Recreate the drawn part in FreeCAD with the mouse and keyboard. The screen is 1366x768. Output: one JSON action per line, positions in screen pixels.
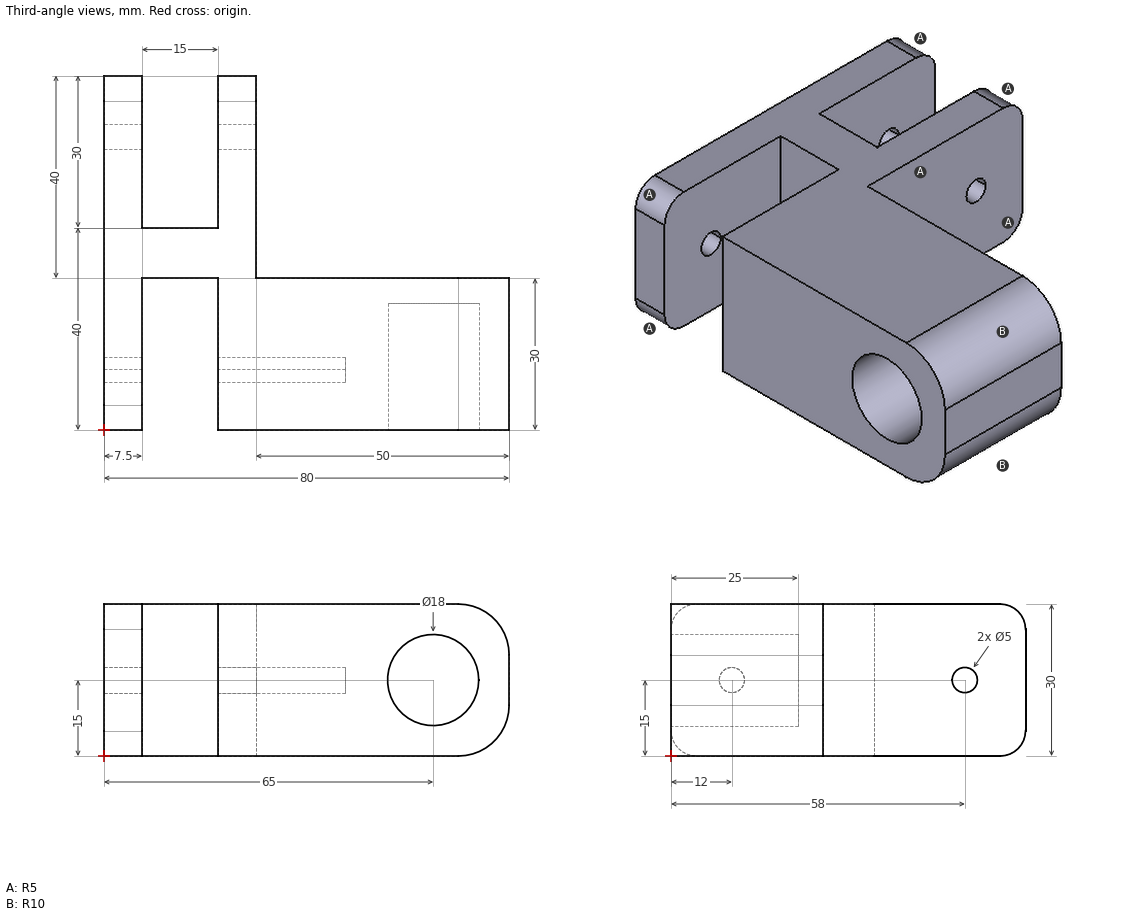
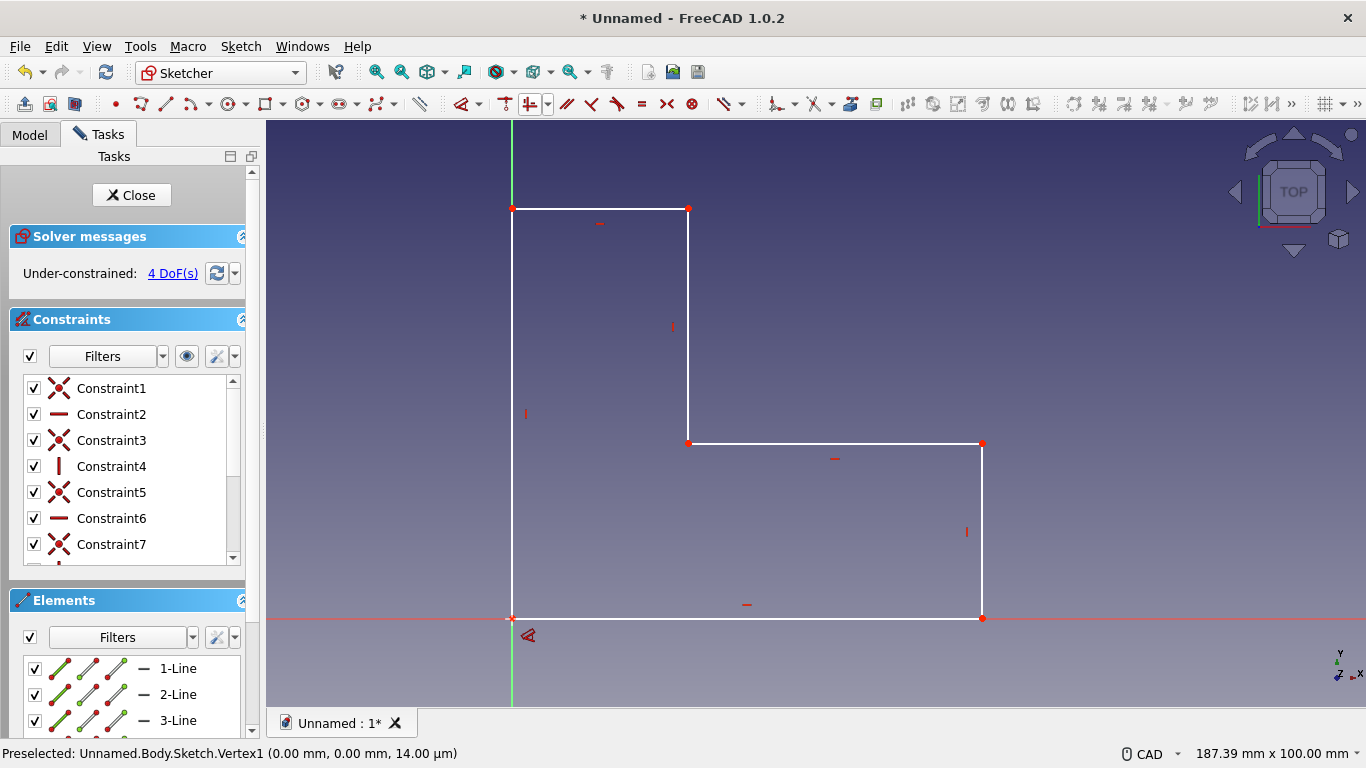
{"action": "left_click", "coordinate": [653, 619]}
{"action": "left_click", "coordinate": [747, 653]}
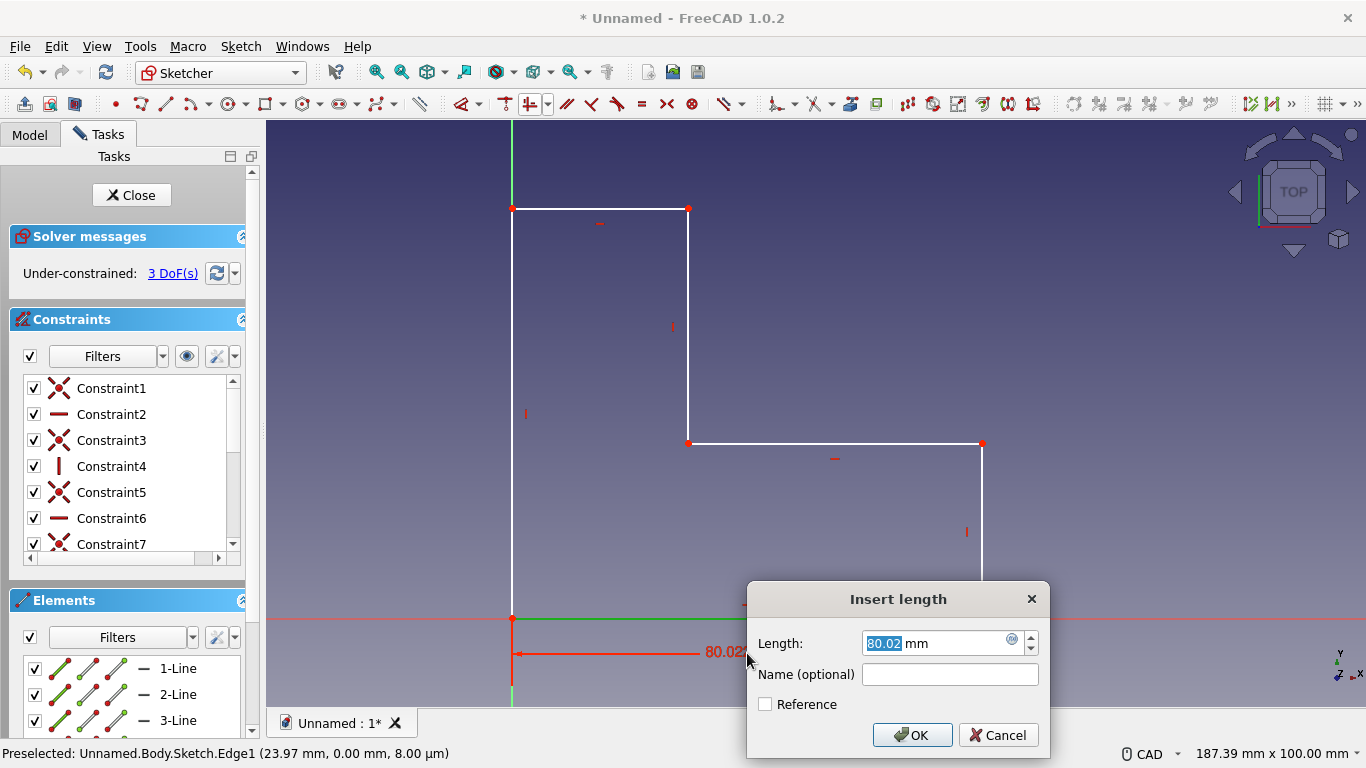
{"action": "type", "text": "80"}
{"action": "key", "text": "Return"}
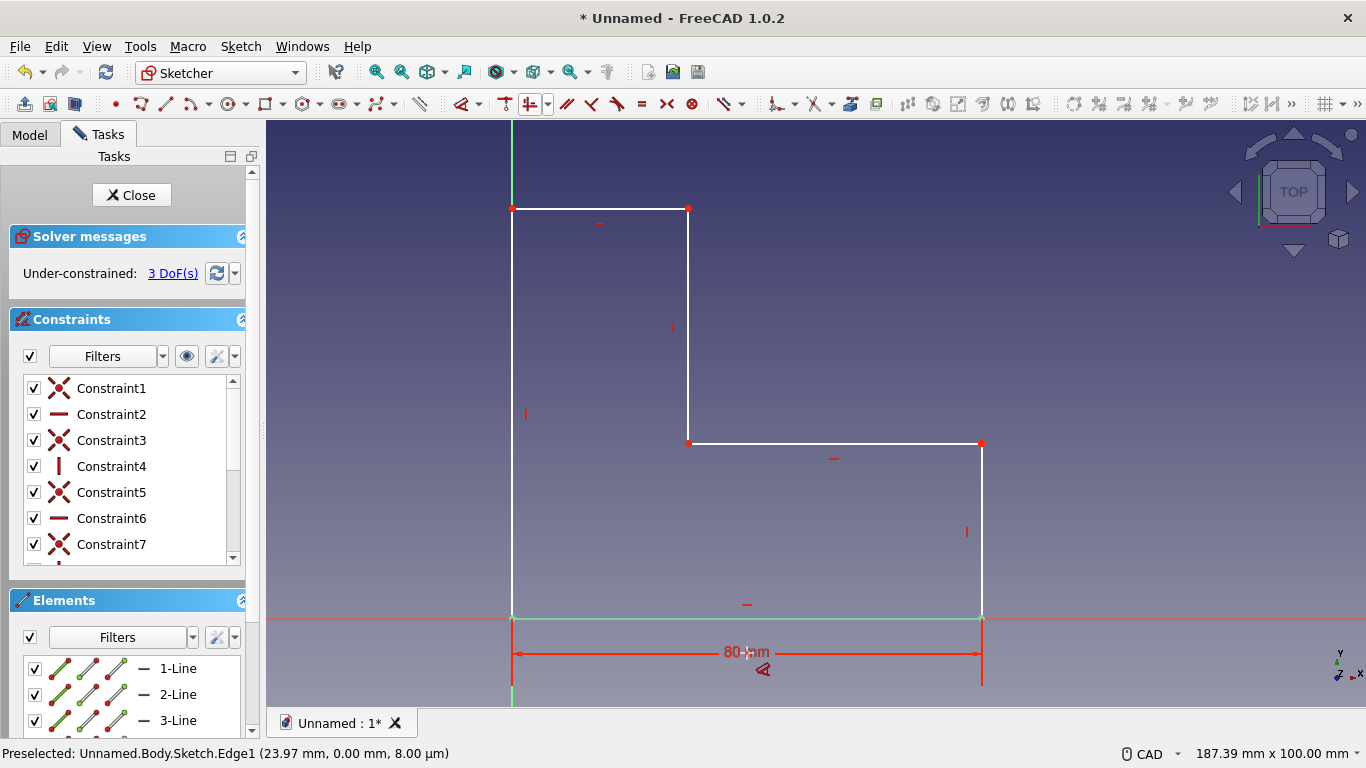
{"action": "left_click", "coordinate": [982, 566]}
{"action": "left_click", "coordinate": [1016, 531]}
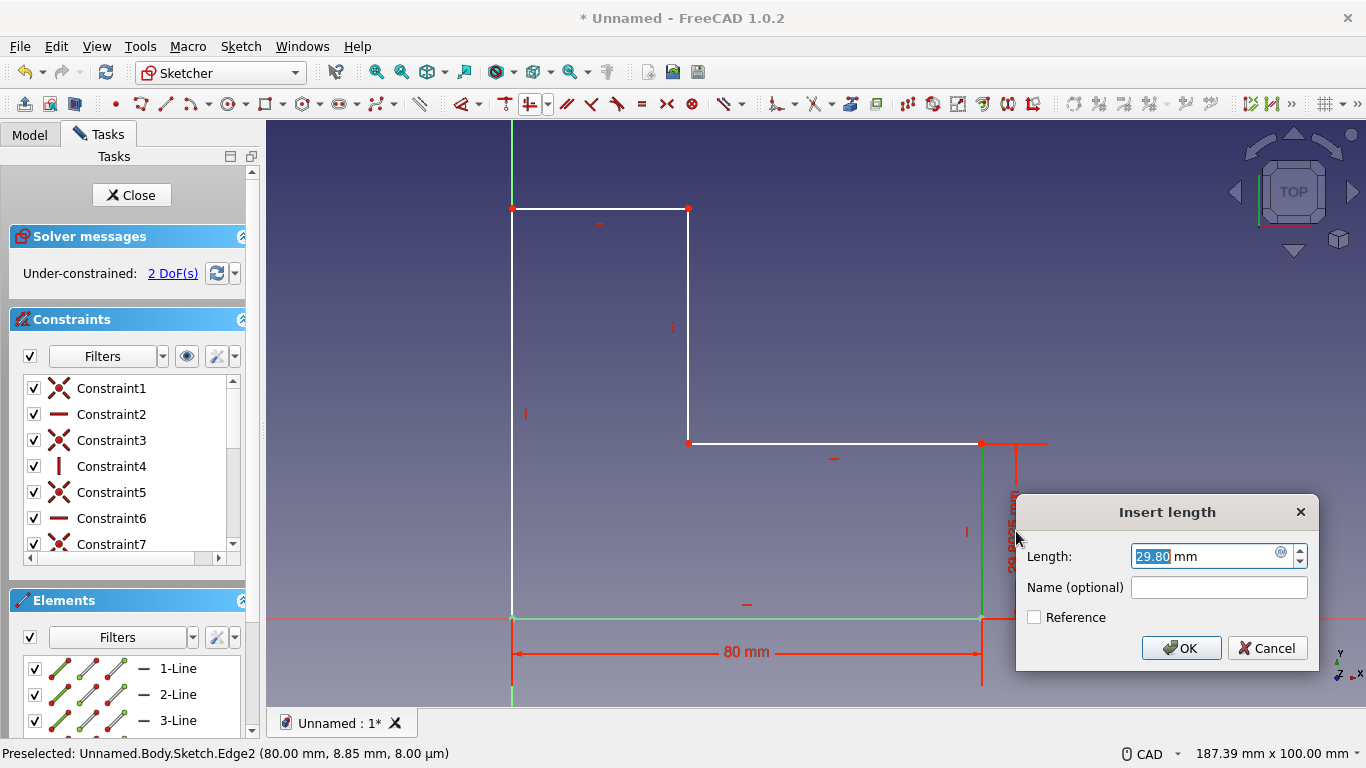
{"action": "type", "text": "30"}
{"action": "key", "text": "Return"}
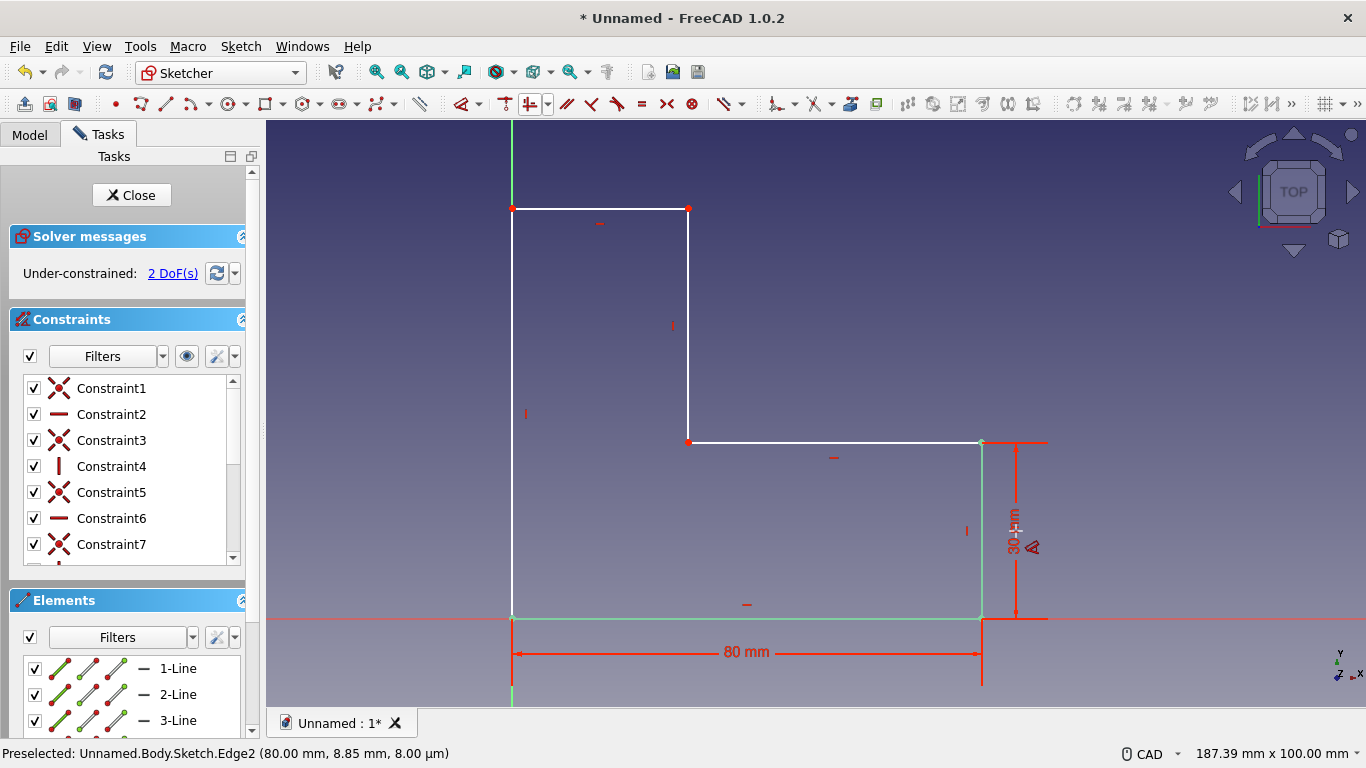
{"action": "left_click", "coordinate": [894, 443]}
{"action": "left_click", "coordinate": [835, 477]}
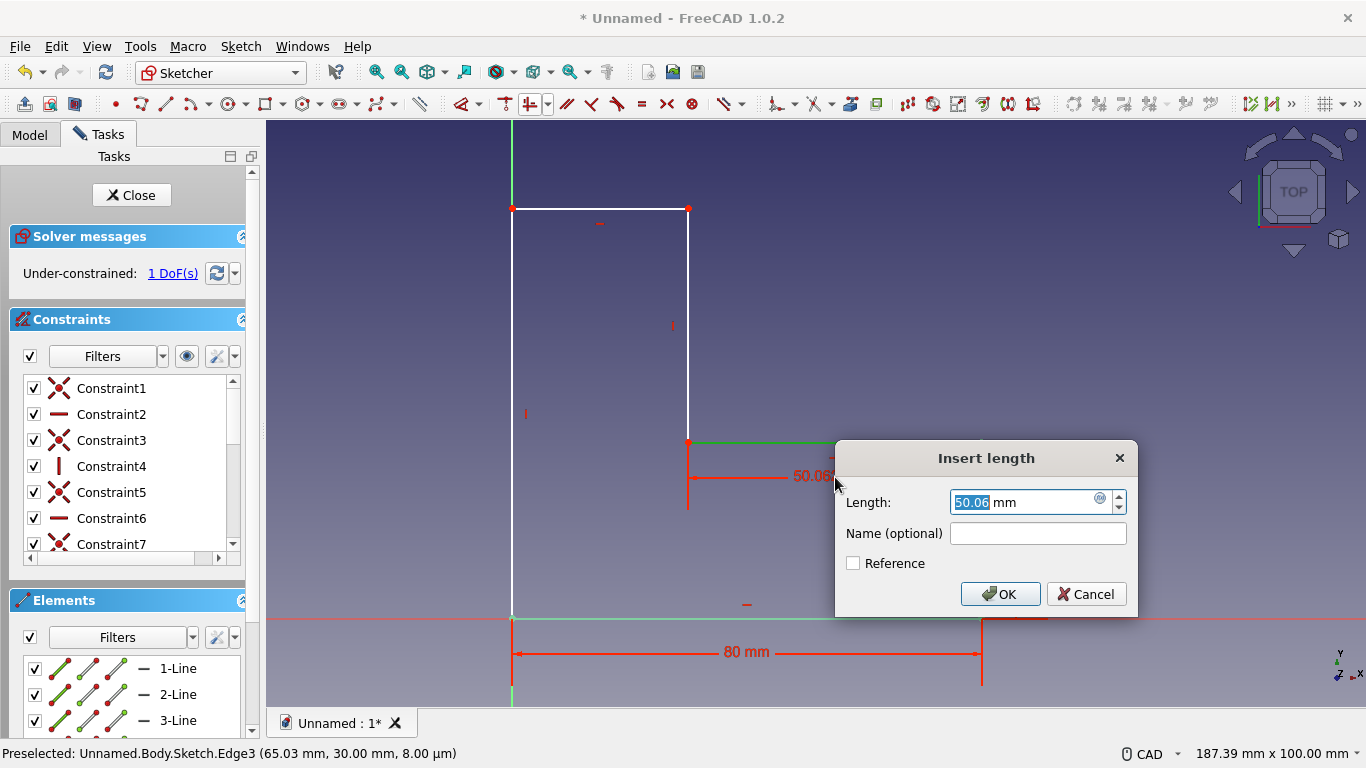
{"action": "type", "text": "50"}
{"action": "key", "text": "Return"}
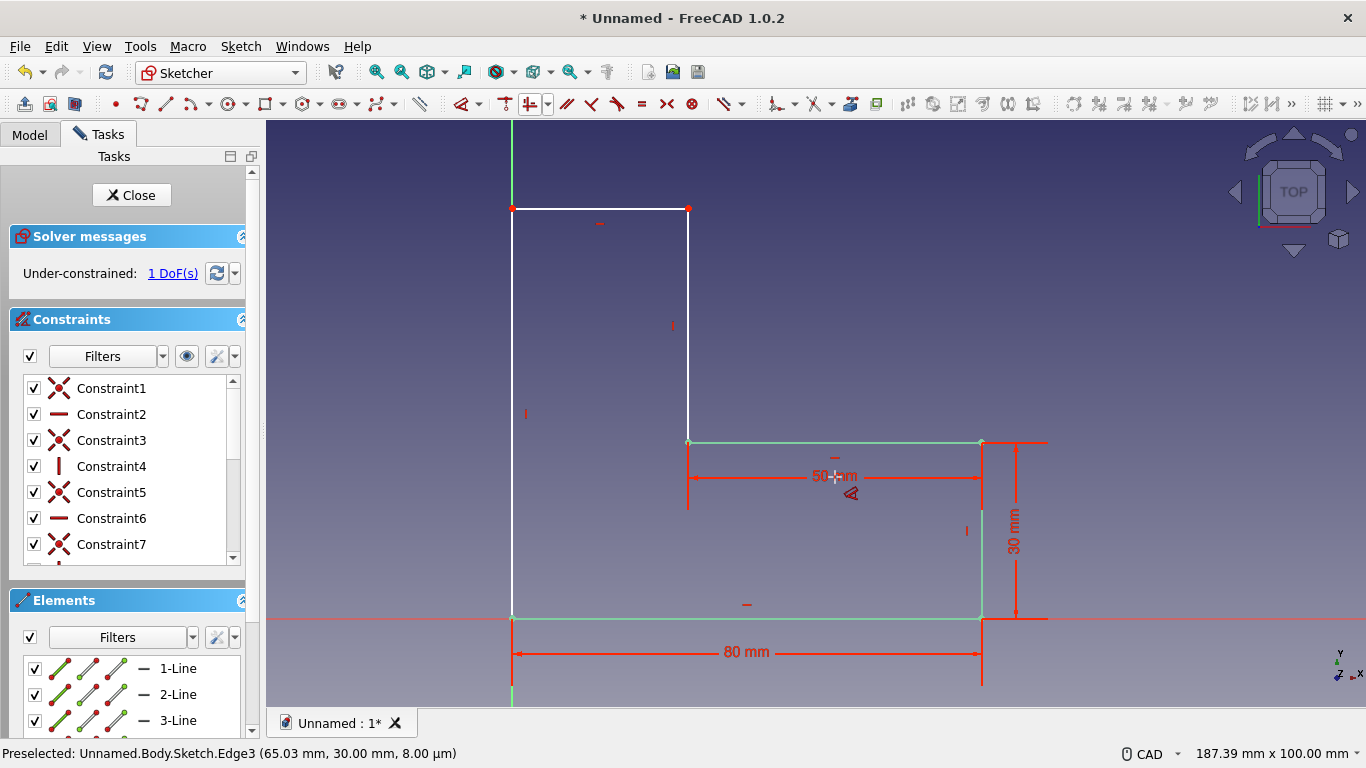
{"action": "left_click", "coordinate": [688, 373]}
{"action": "left_click", "coordinate": [654, 326]}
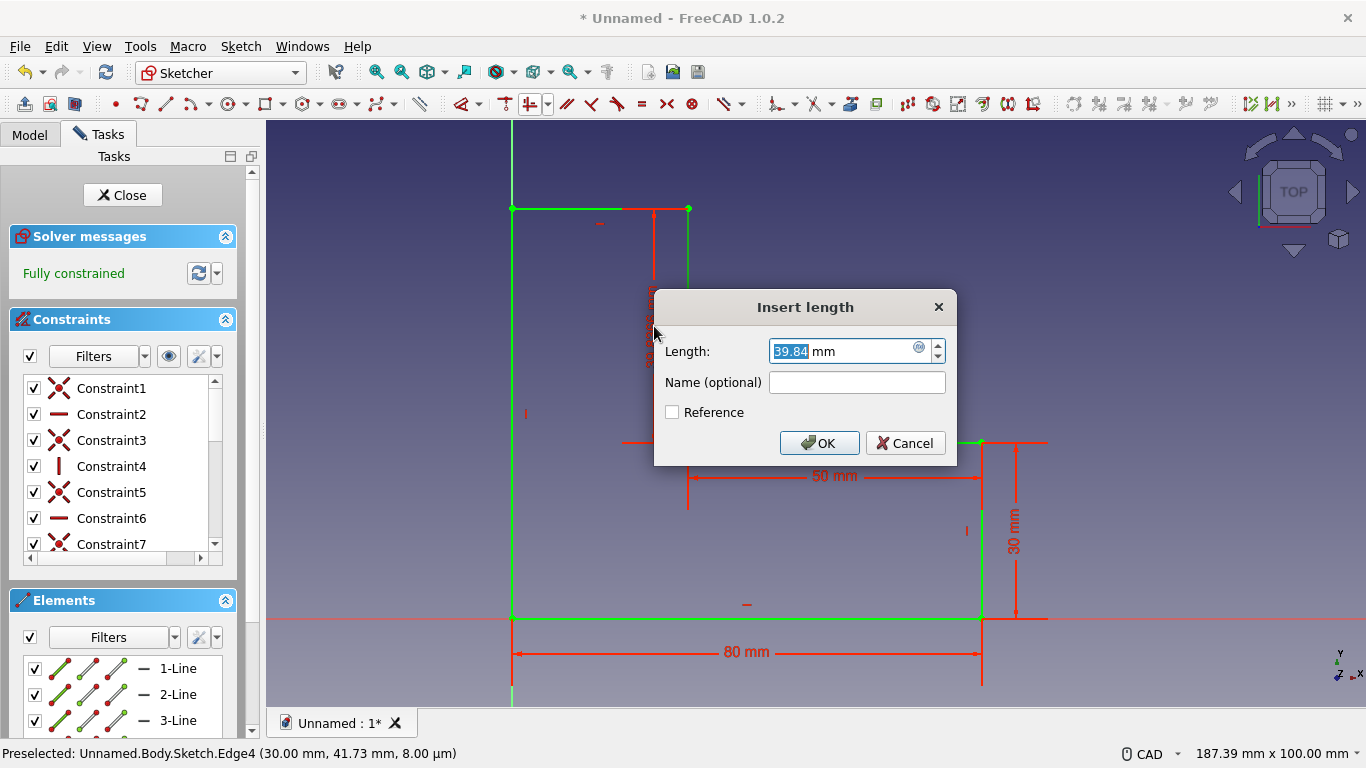
{"action": "type", "text": "40"}
{"action": "key", "text": "Return"}
{"action": "key", "text": "Escape"}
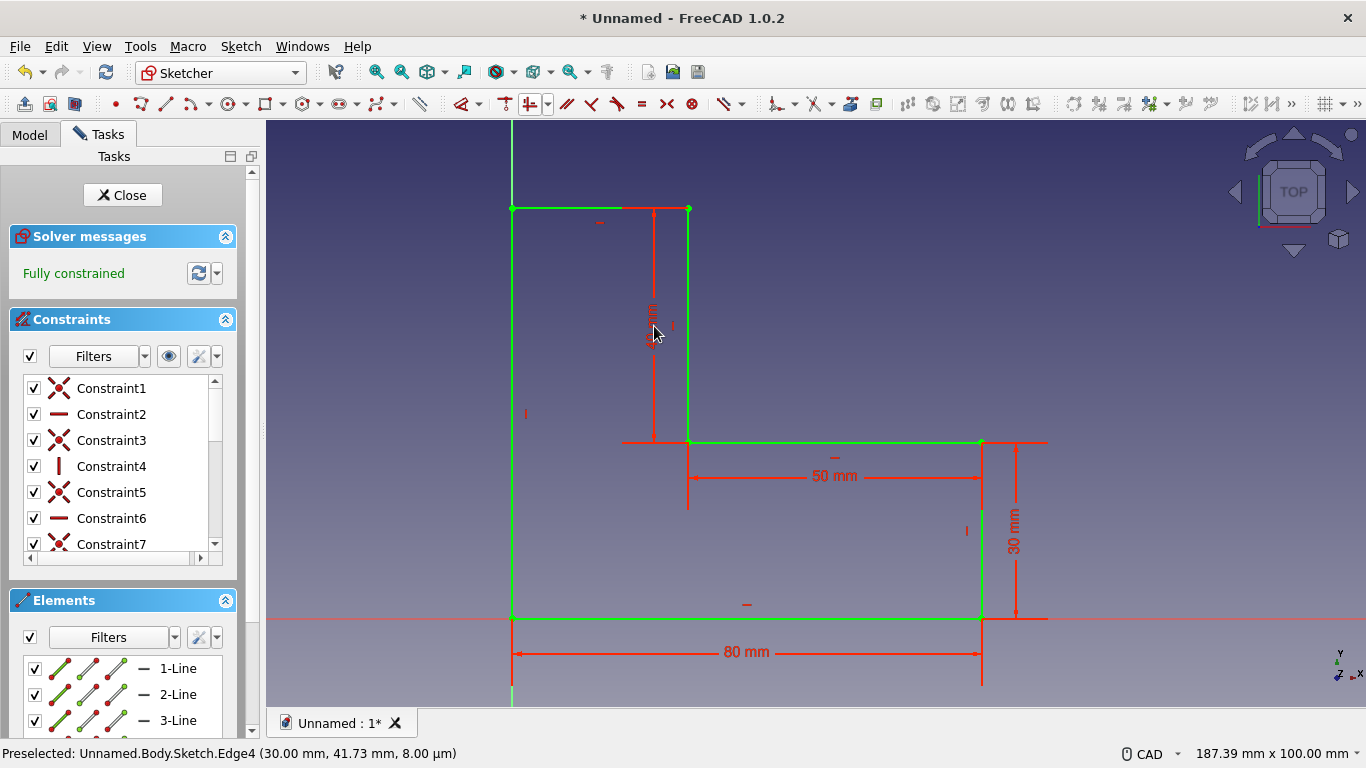
{"action": "left_click", "coordinate": [123, 195]}